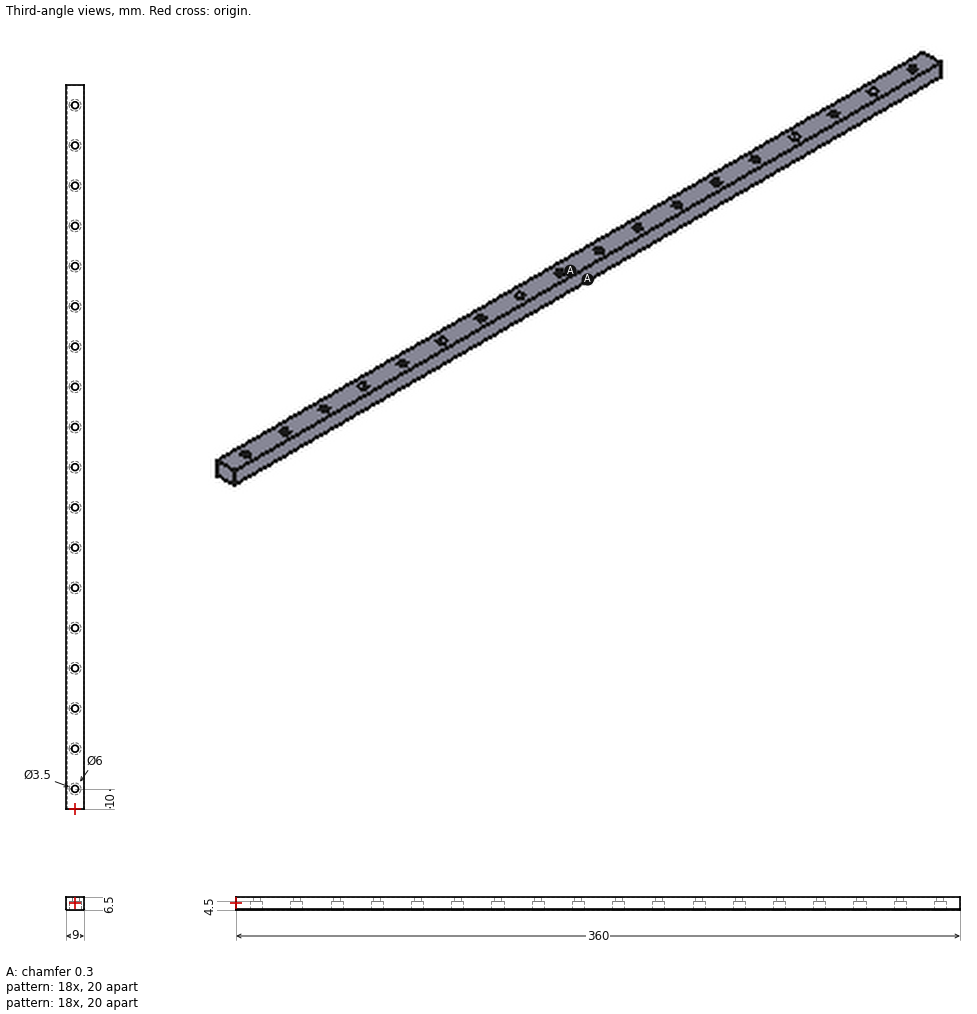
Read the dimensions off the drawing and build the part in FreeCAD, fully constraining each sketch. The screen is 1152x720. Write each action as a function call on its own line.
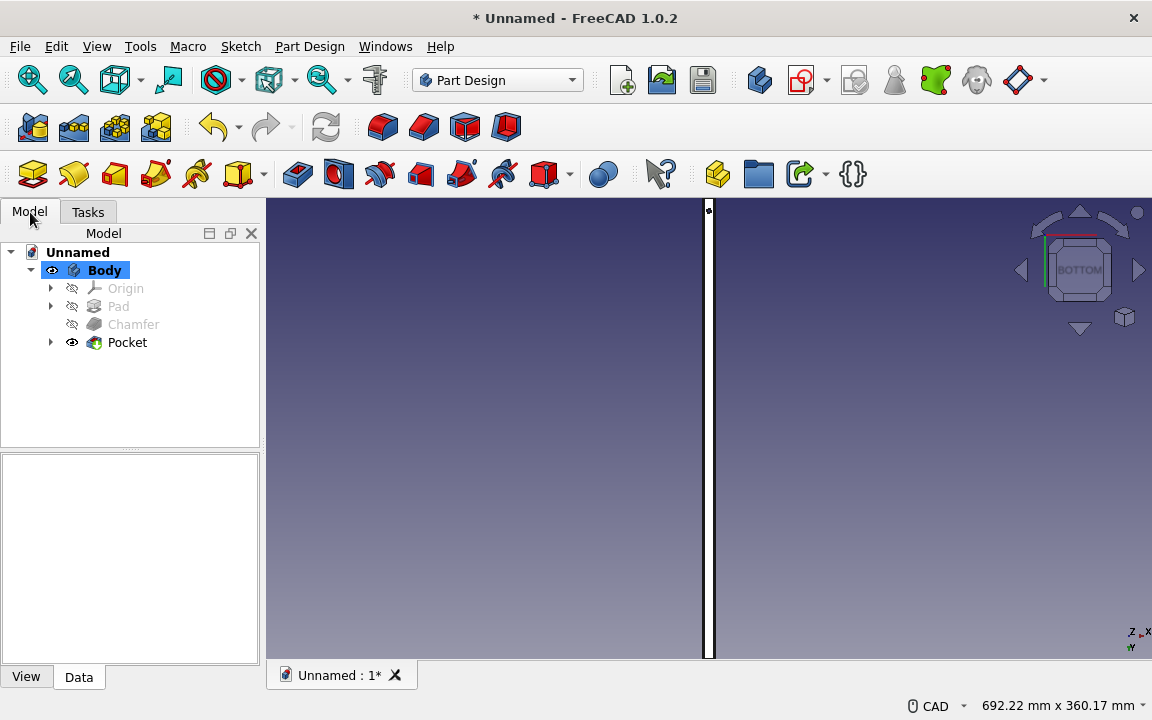
click(117, 342)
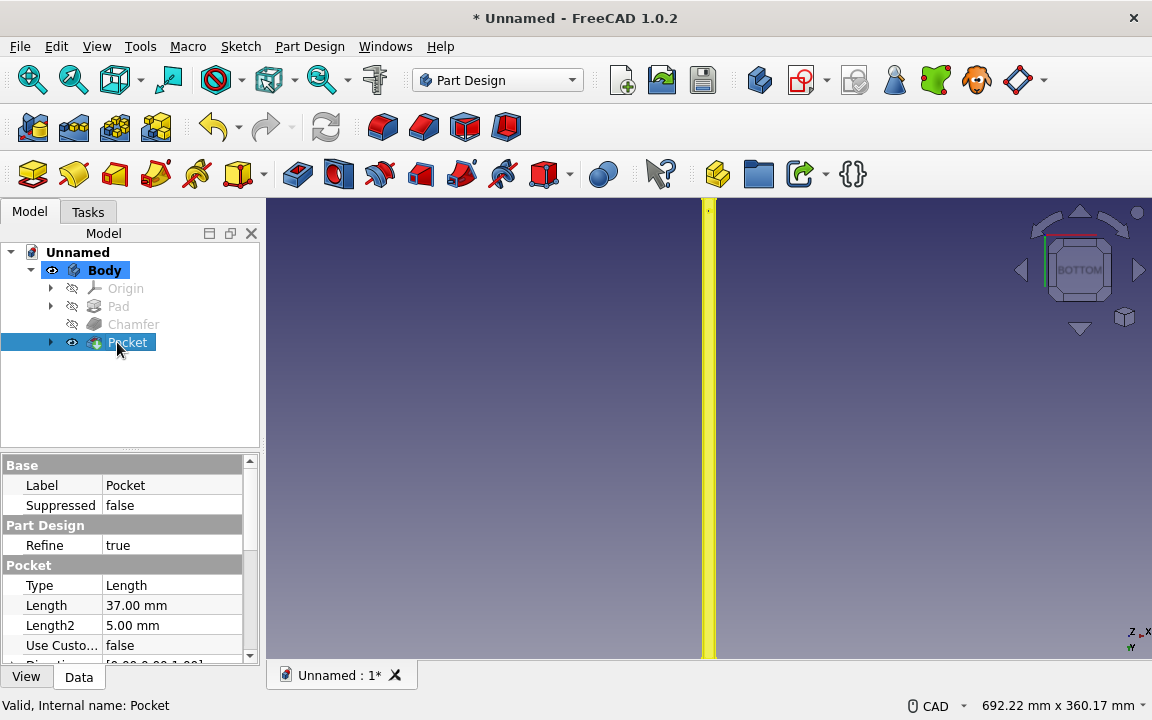
click(74, 128)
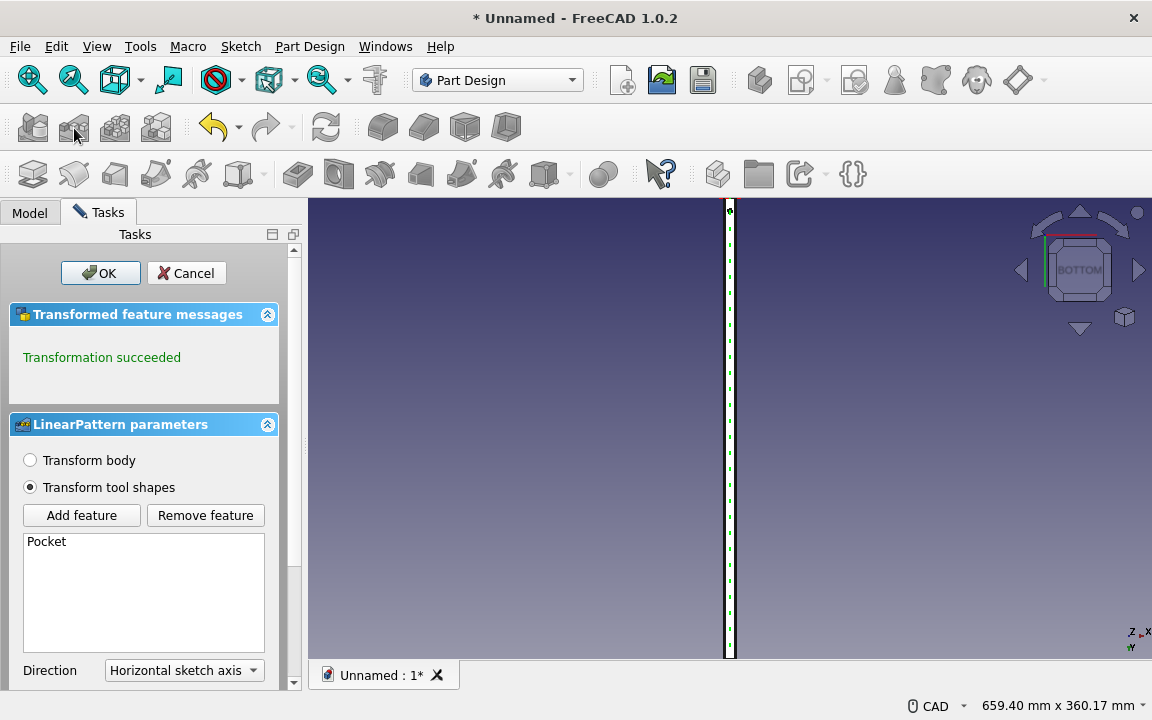
click(185, 670)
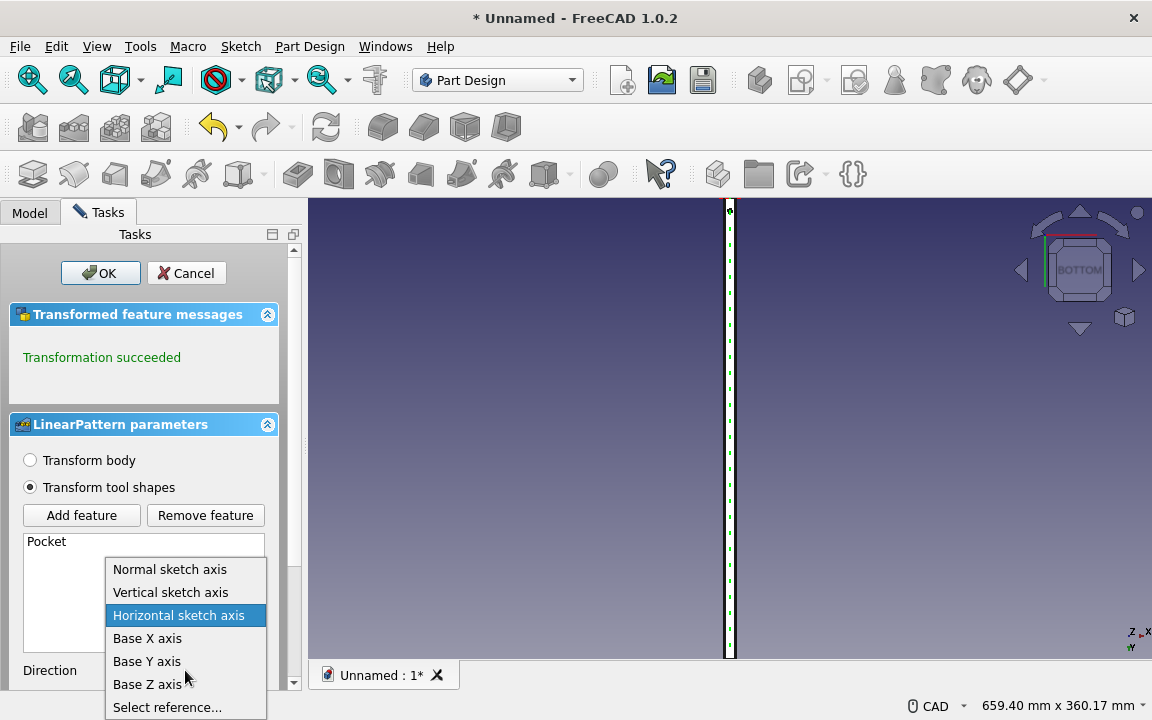
click(184, 662)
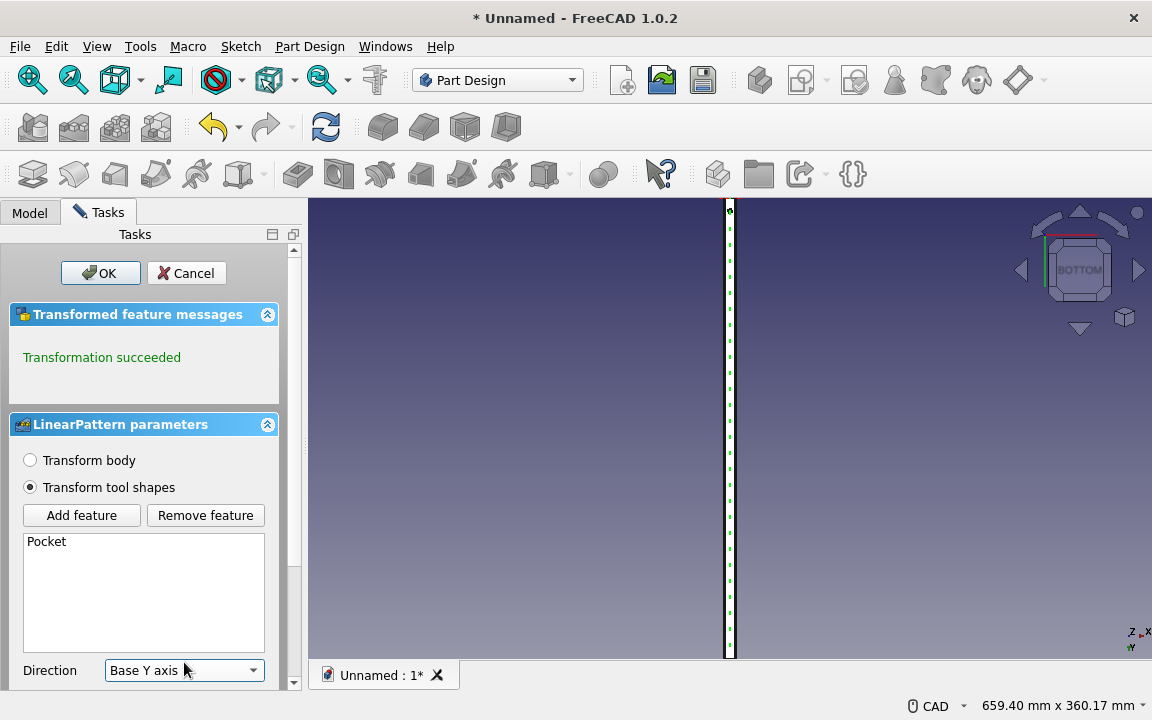
scroll(294, 467, down, 2)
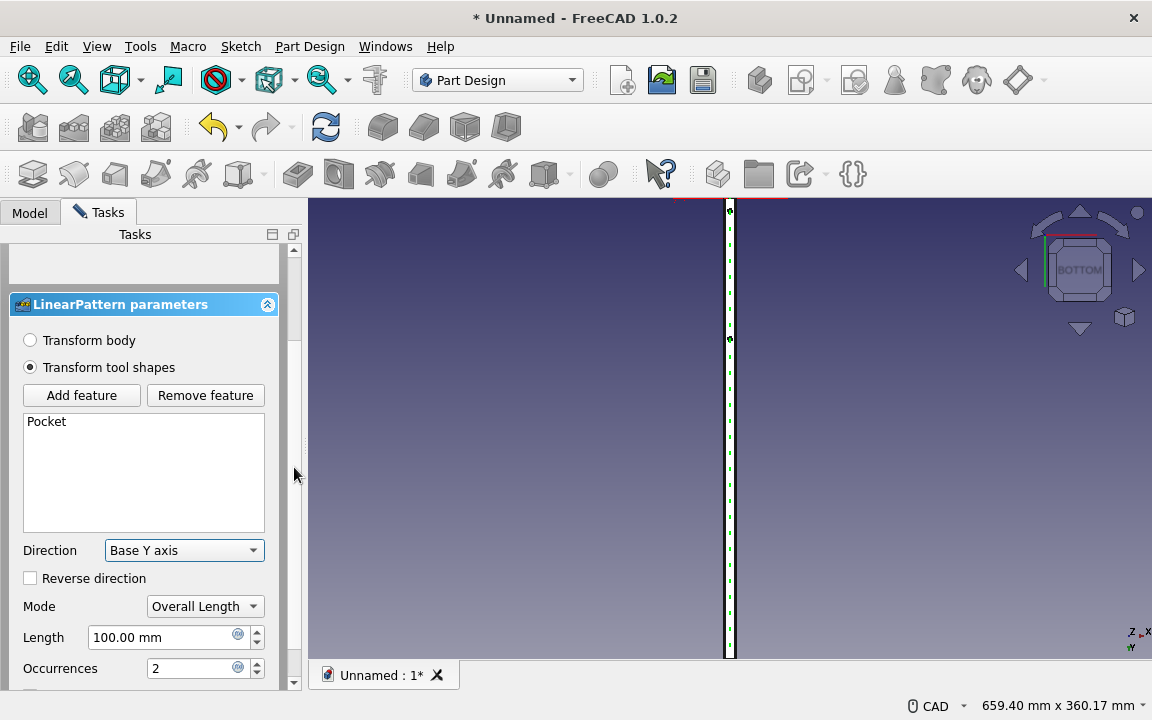
click(206, 606)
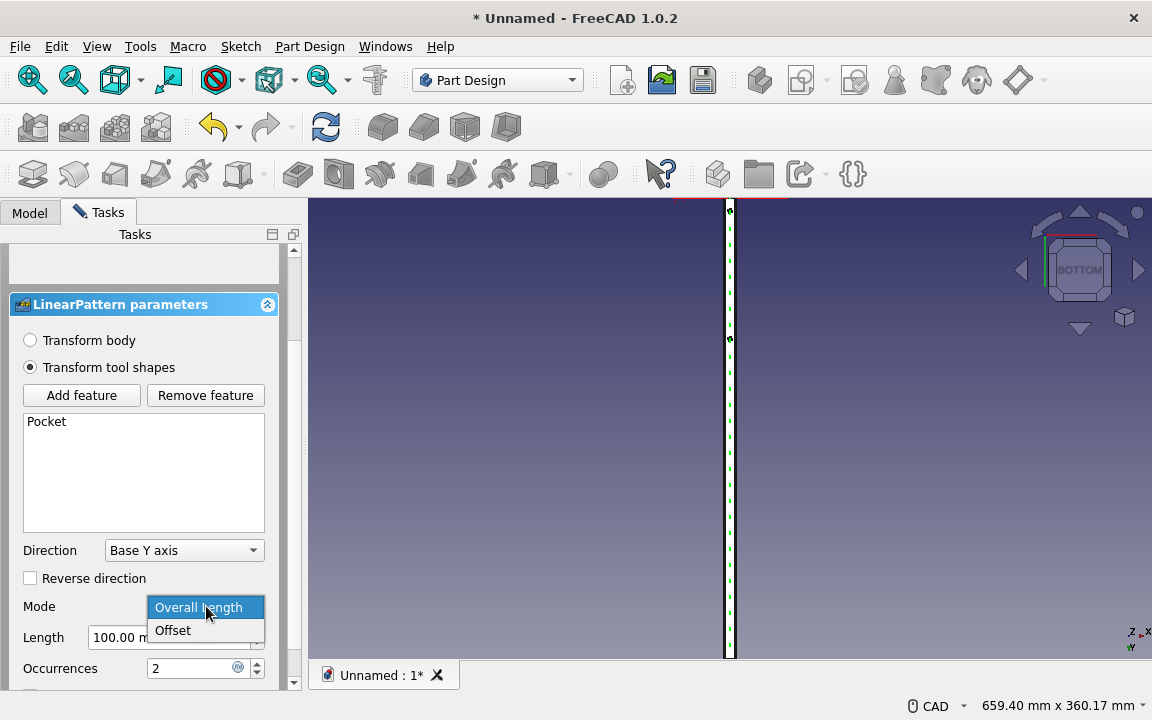
click(204, 630)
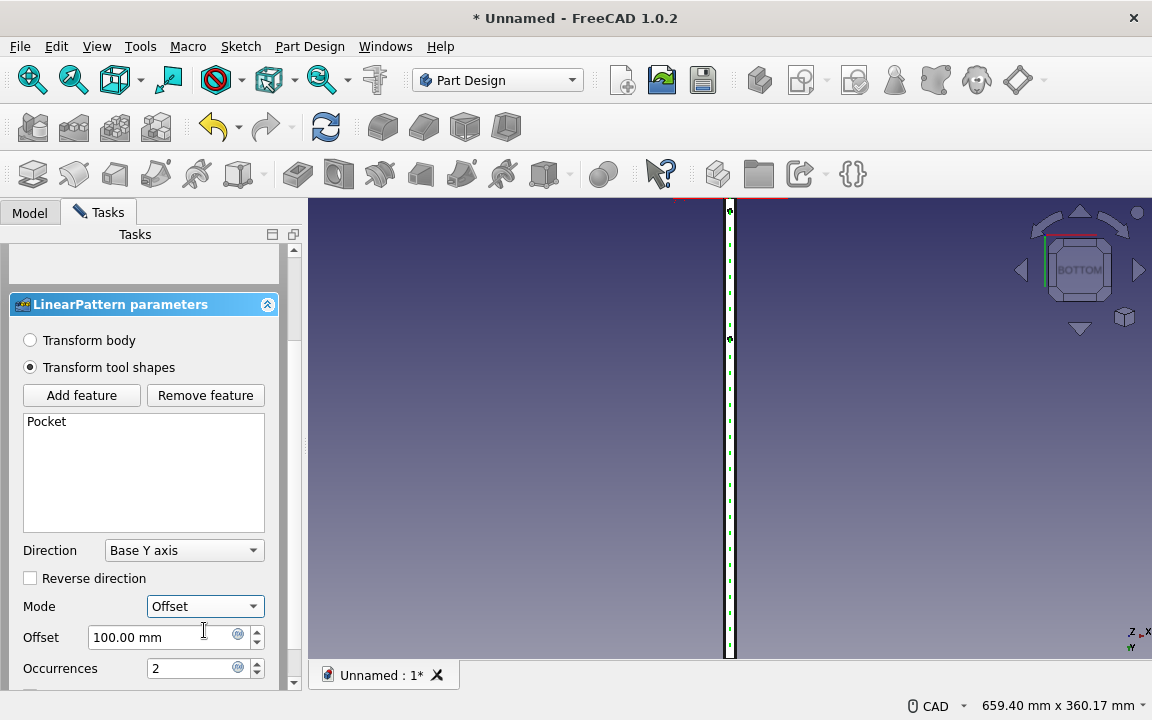
triple_click(170, 638)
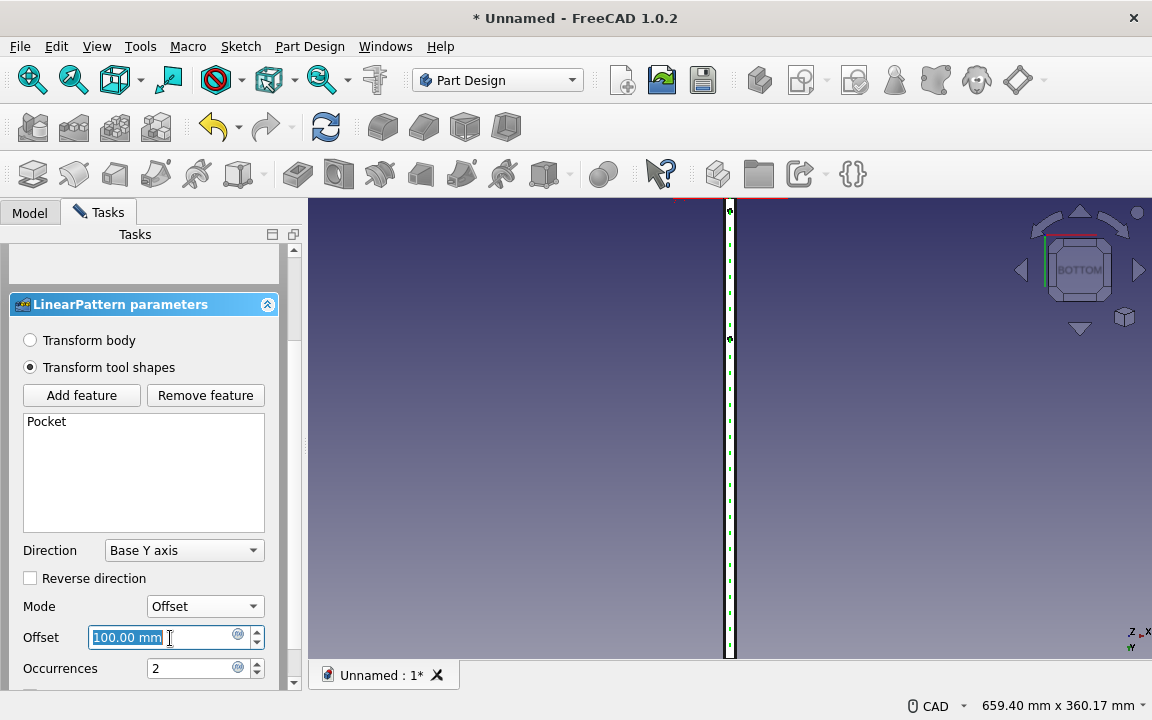
text(20)
key(Tab)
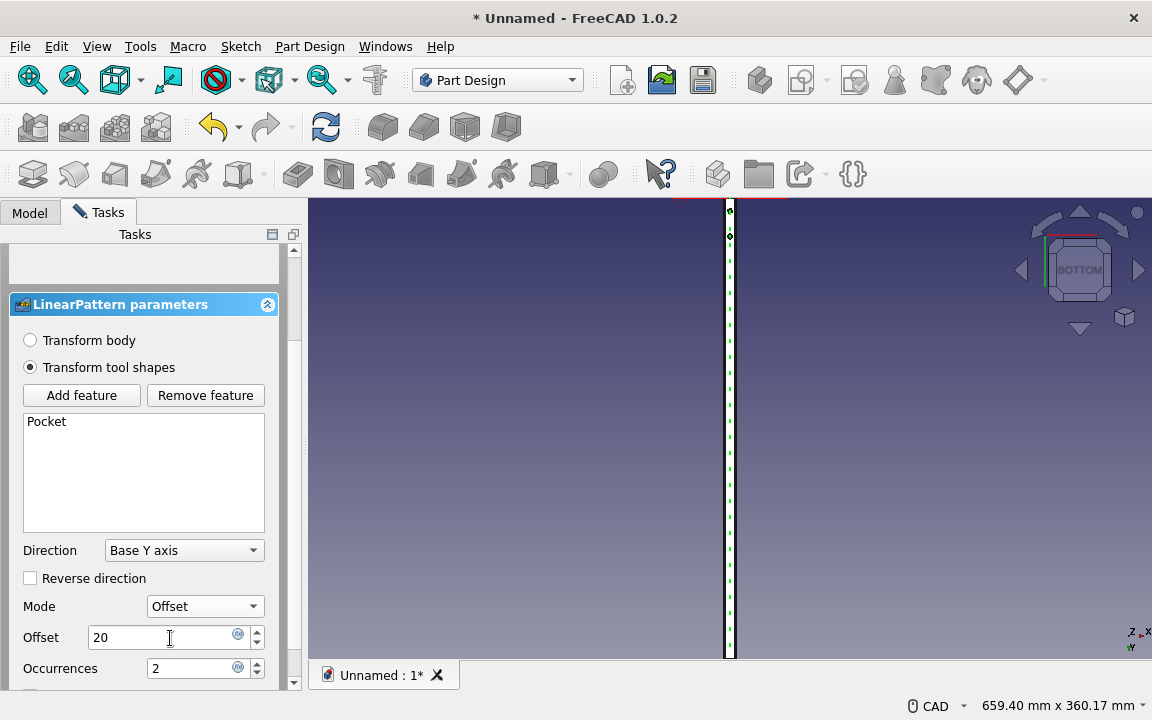
triple_click(199, 668)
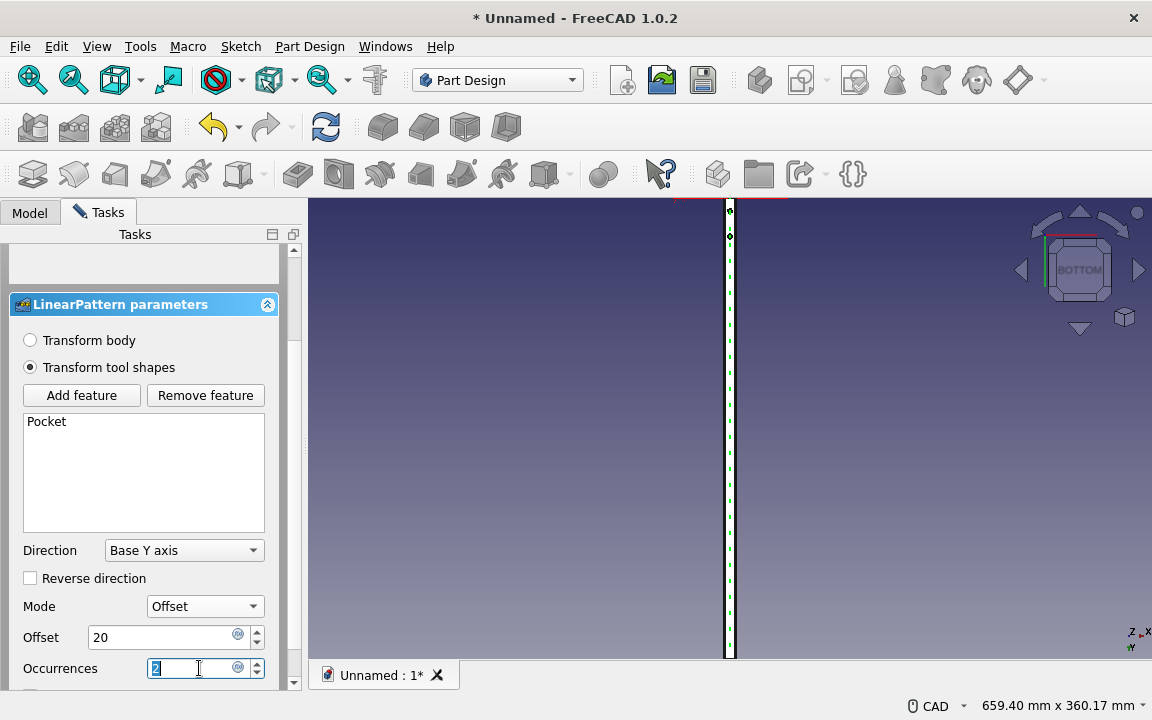
text(18)
key(Tab)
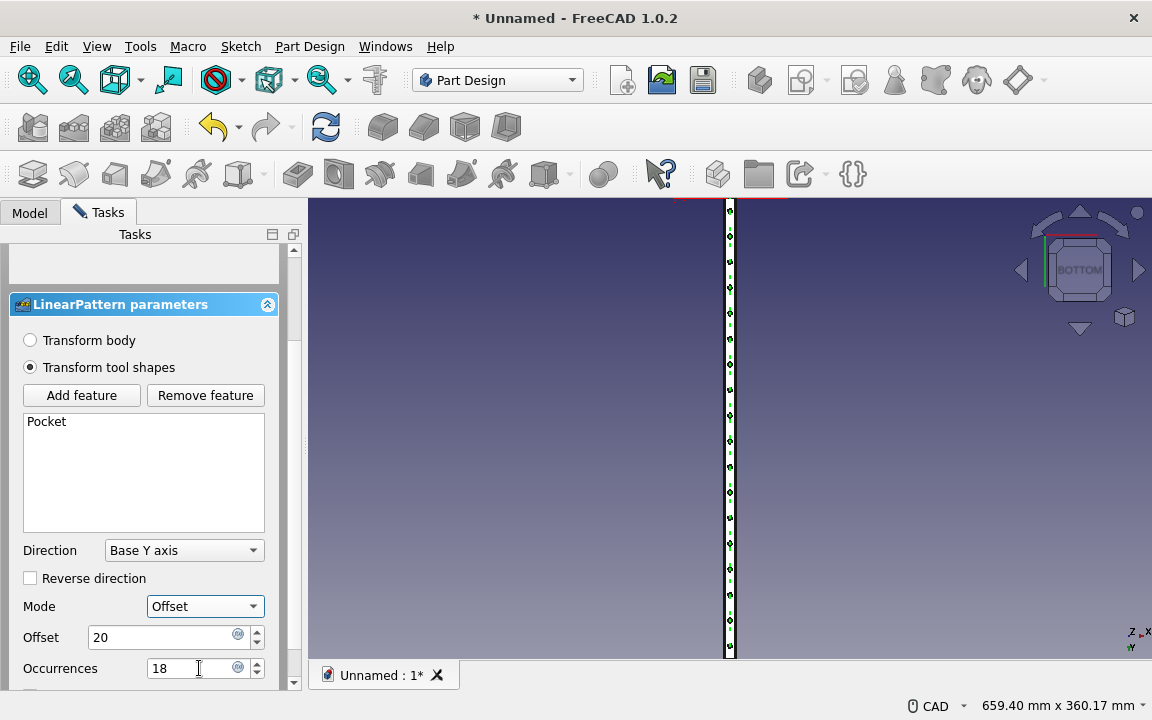
scroll(294, 467, up, 3)